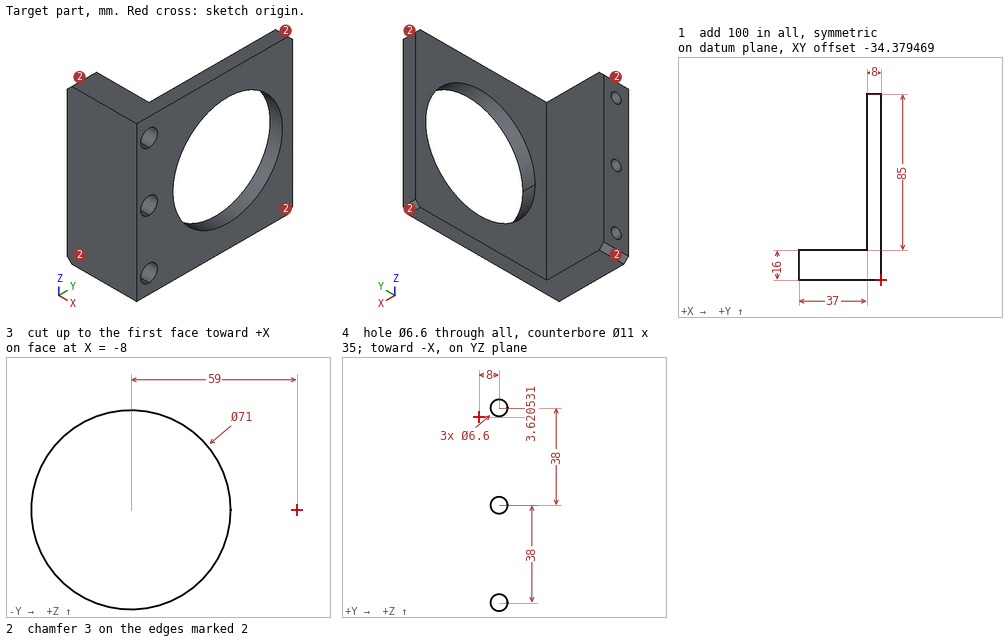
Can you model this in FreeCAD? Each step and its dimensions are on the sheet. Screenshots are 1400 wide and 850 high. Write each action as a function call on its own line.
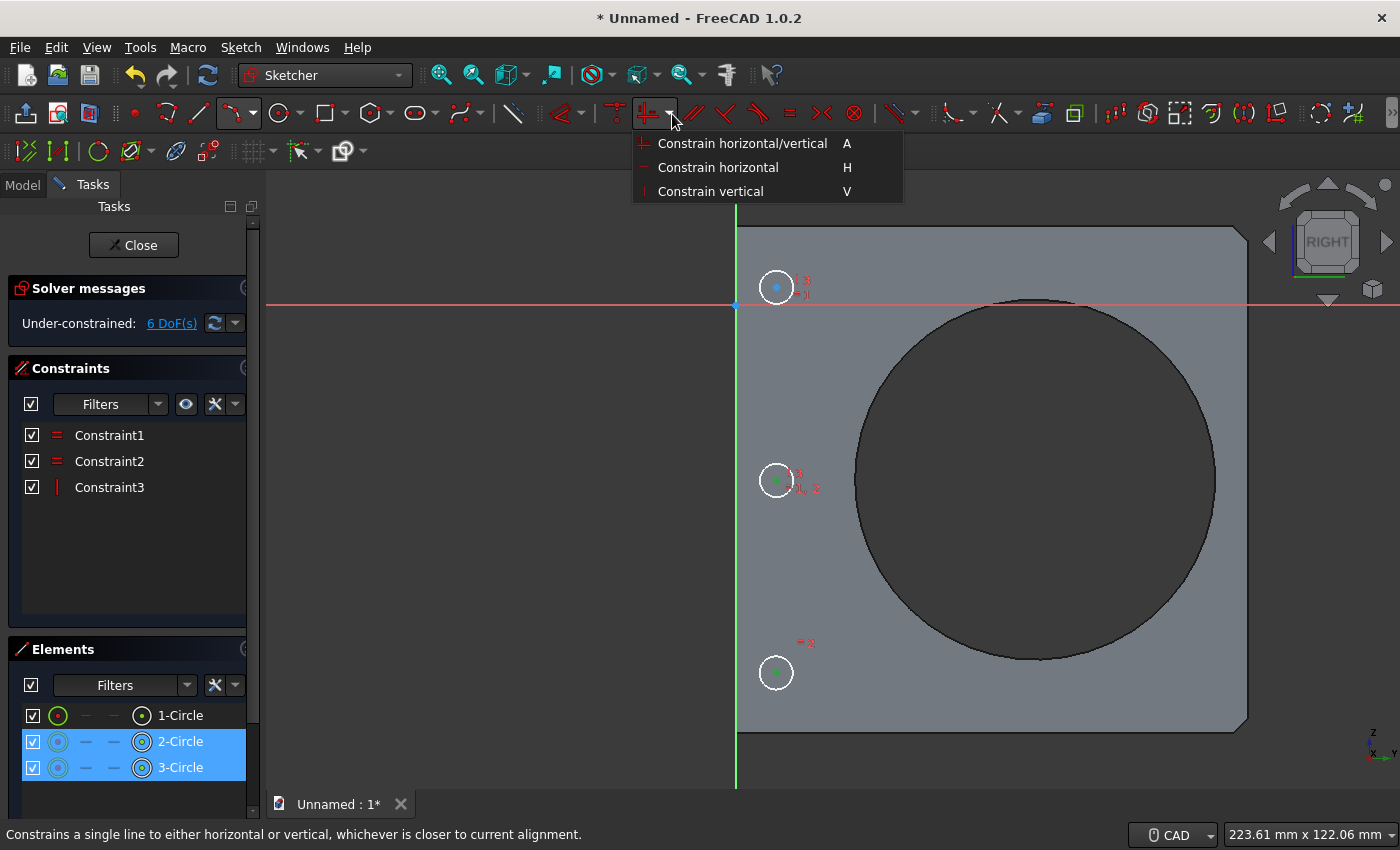
click(768, 191)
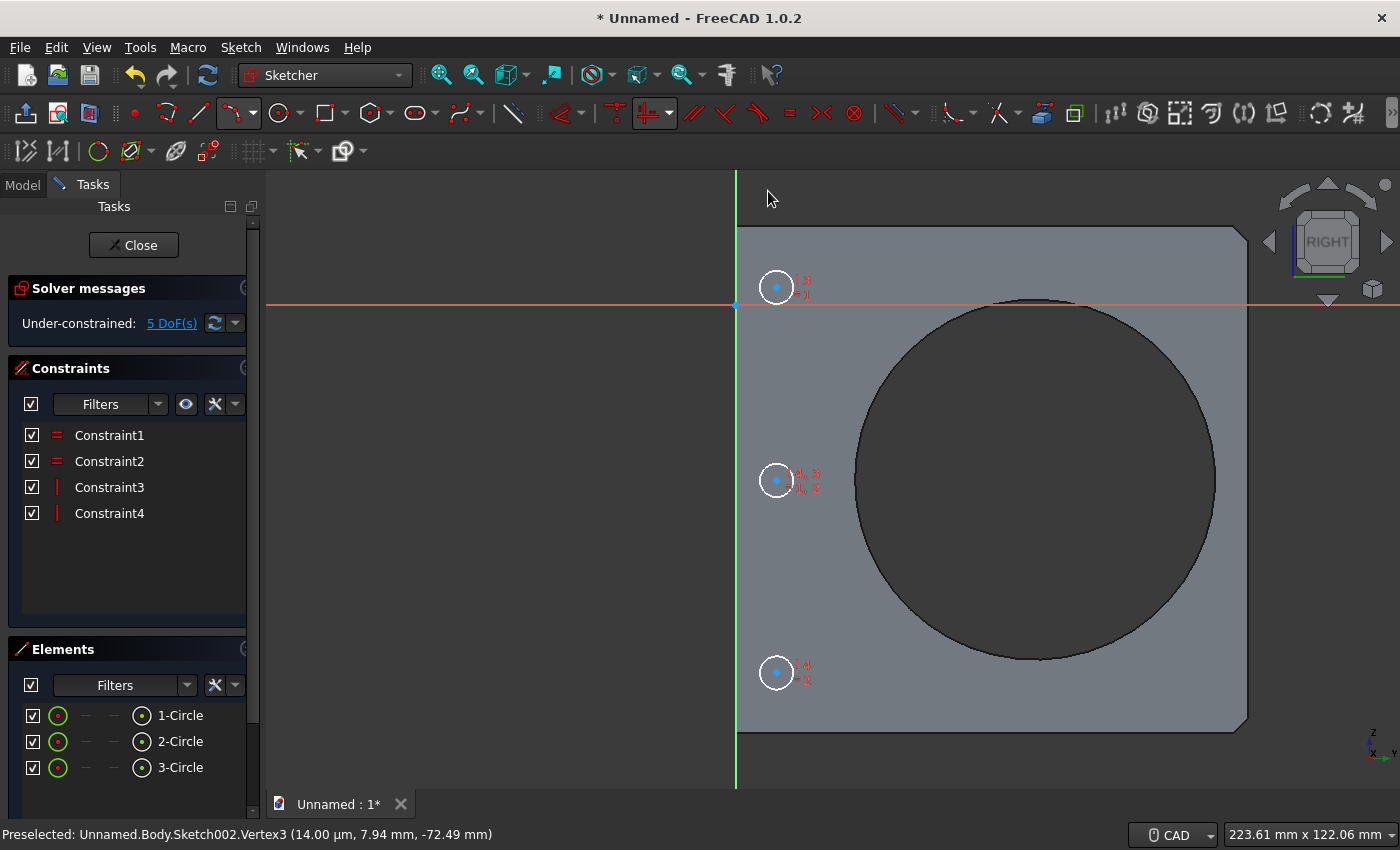
click(560, 114)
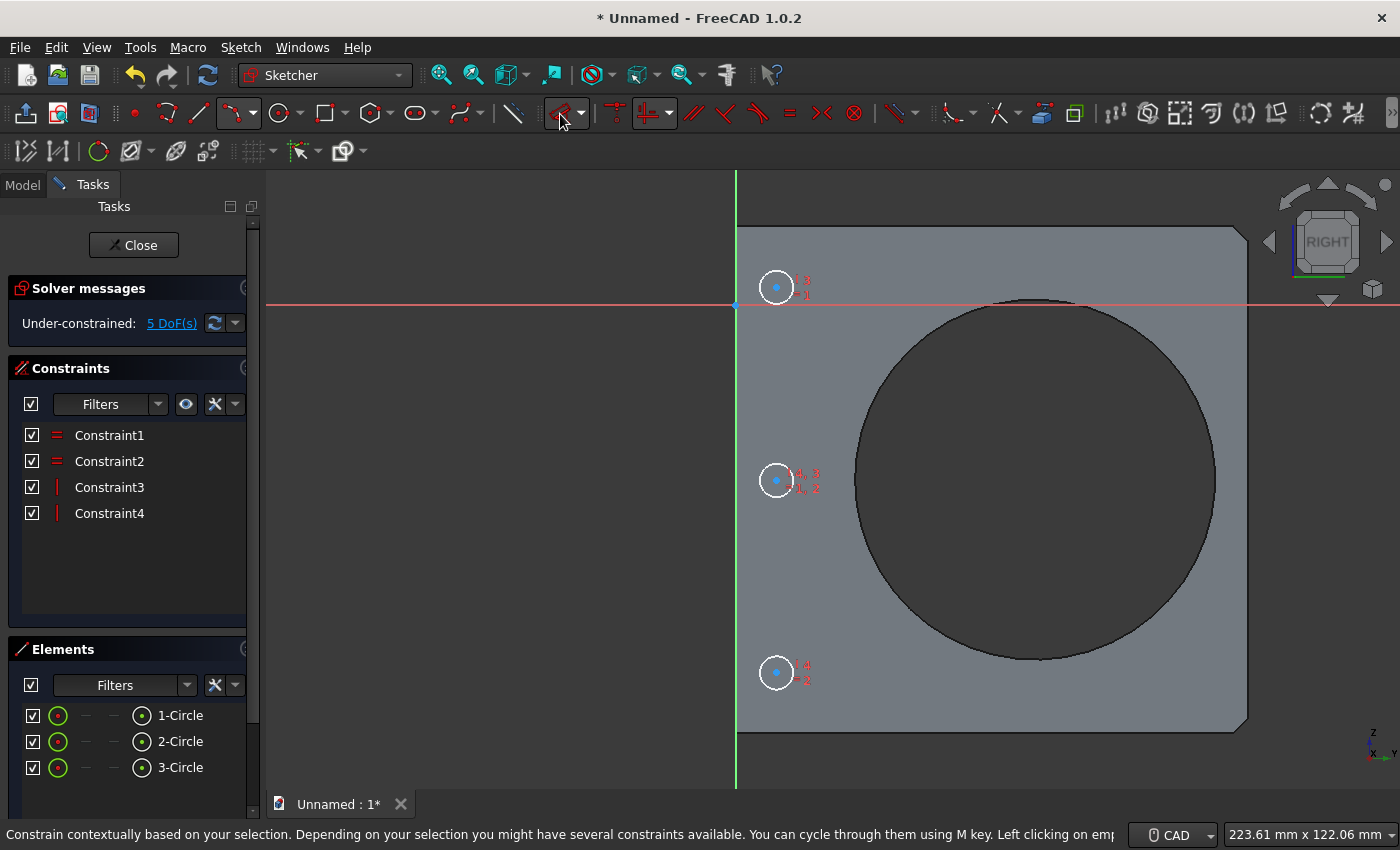
click(788, 276)
click(811, 253)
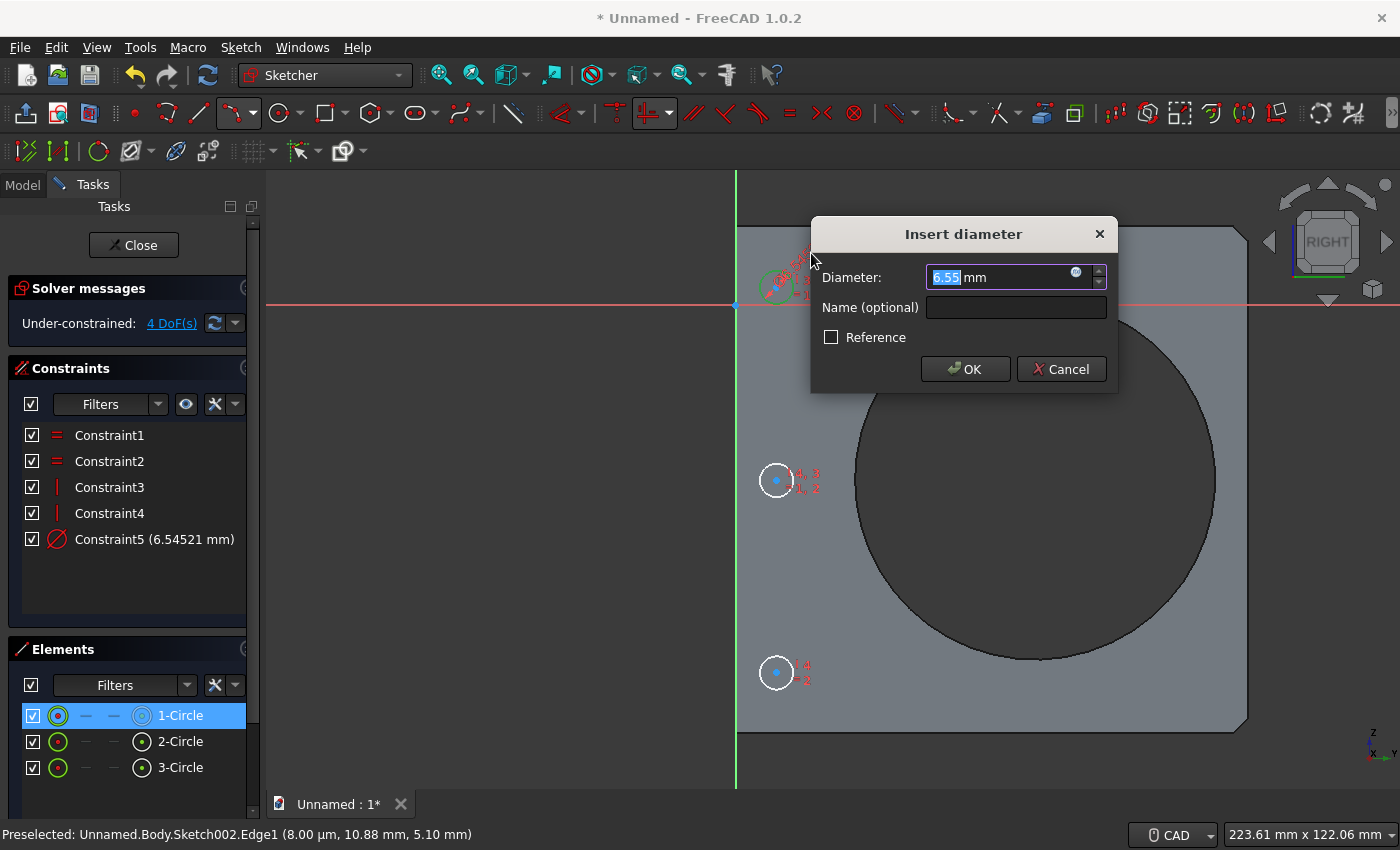
text(6.6)
key(Return)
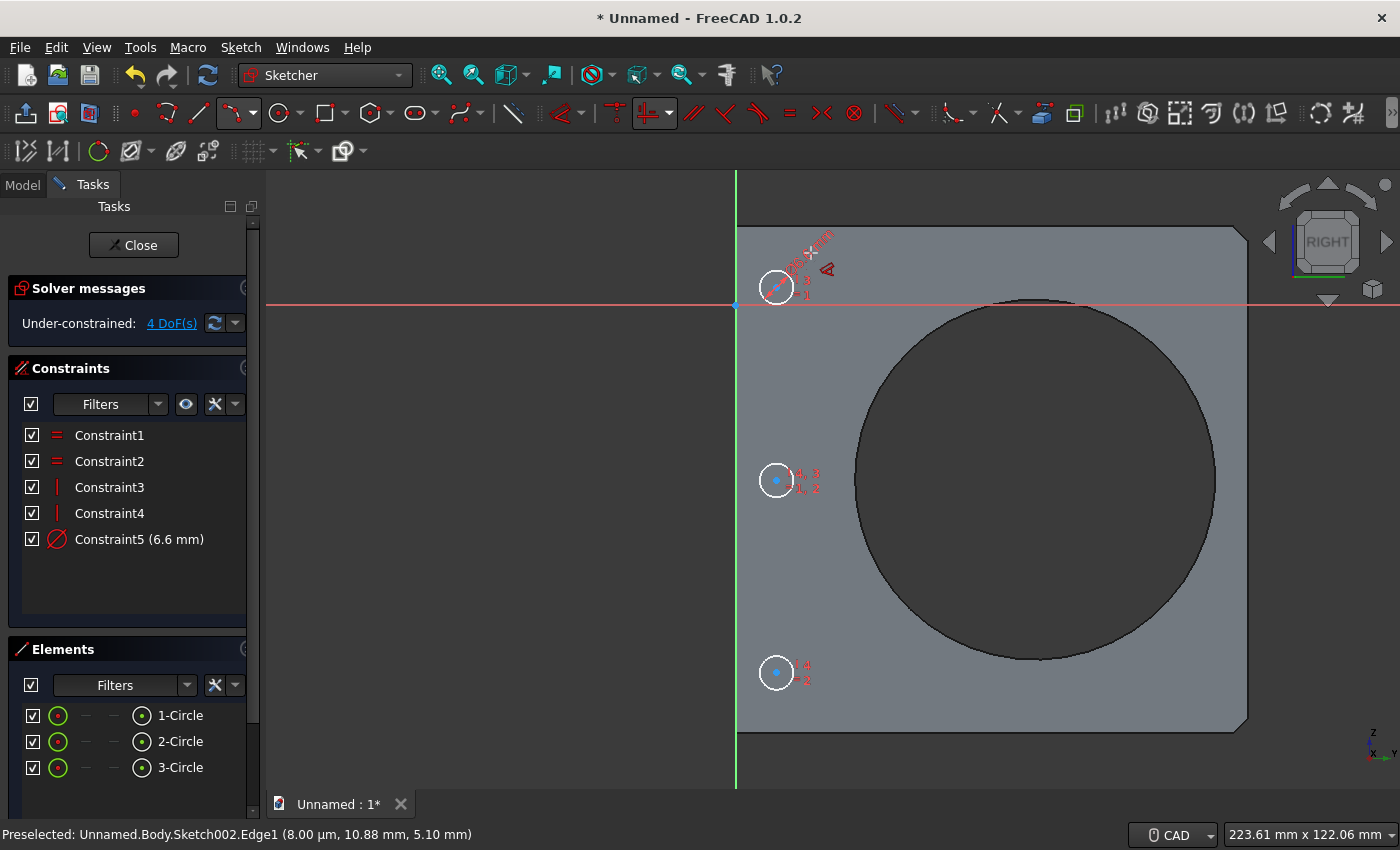
click(777, 287)
click(756, 339)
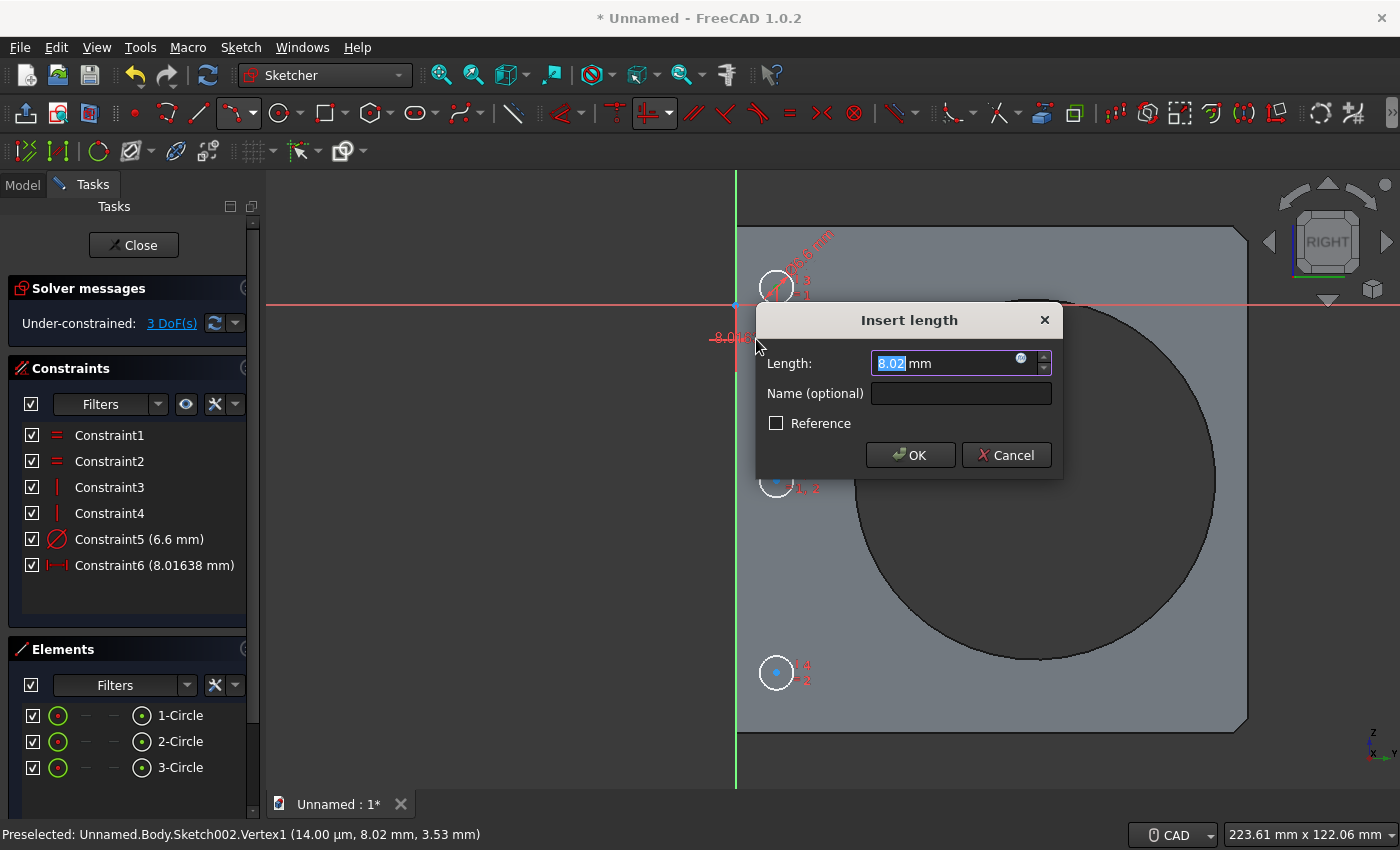
text(8)
key(Return)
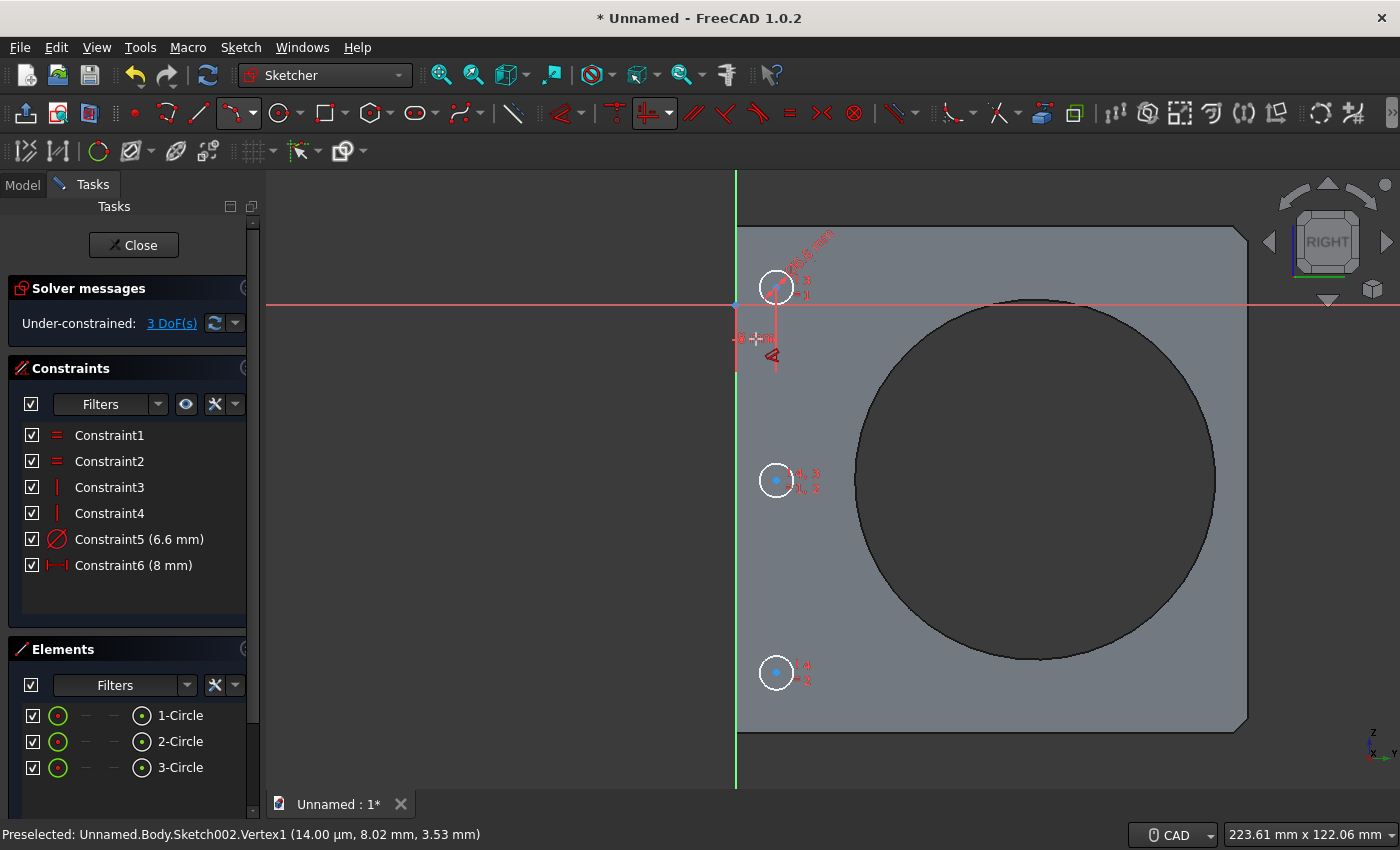
click(776, 287)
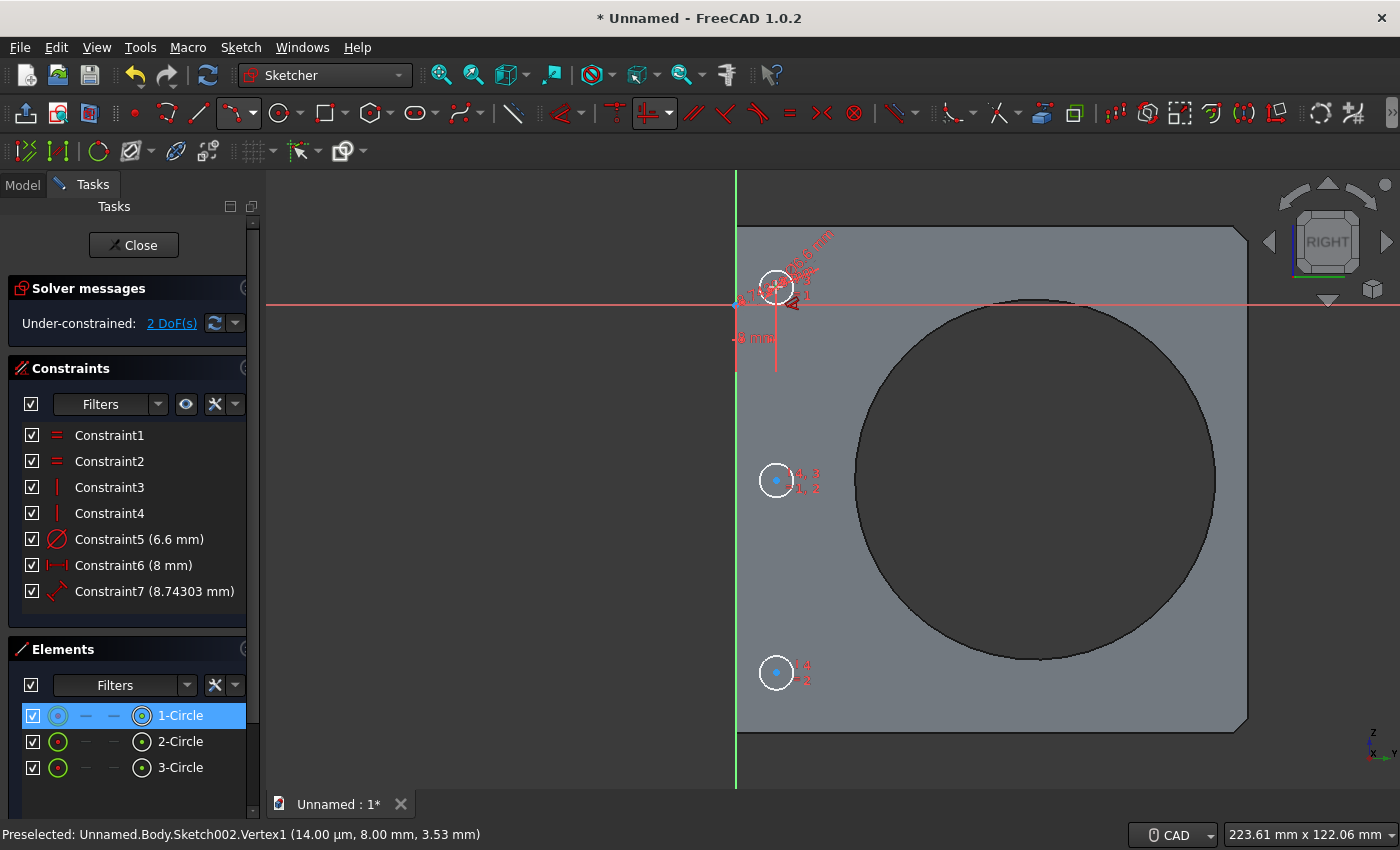
click(776, 480)
click(810, 384)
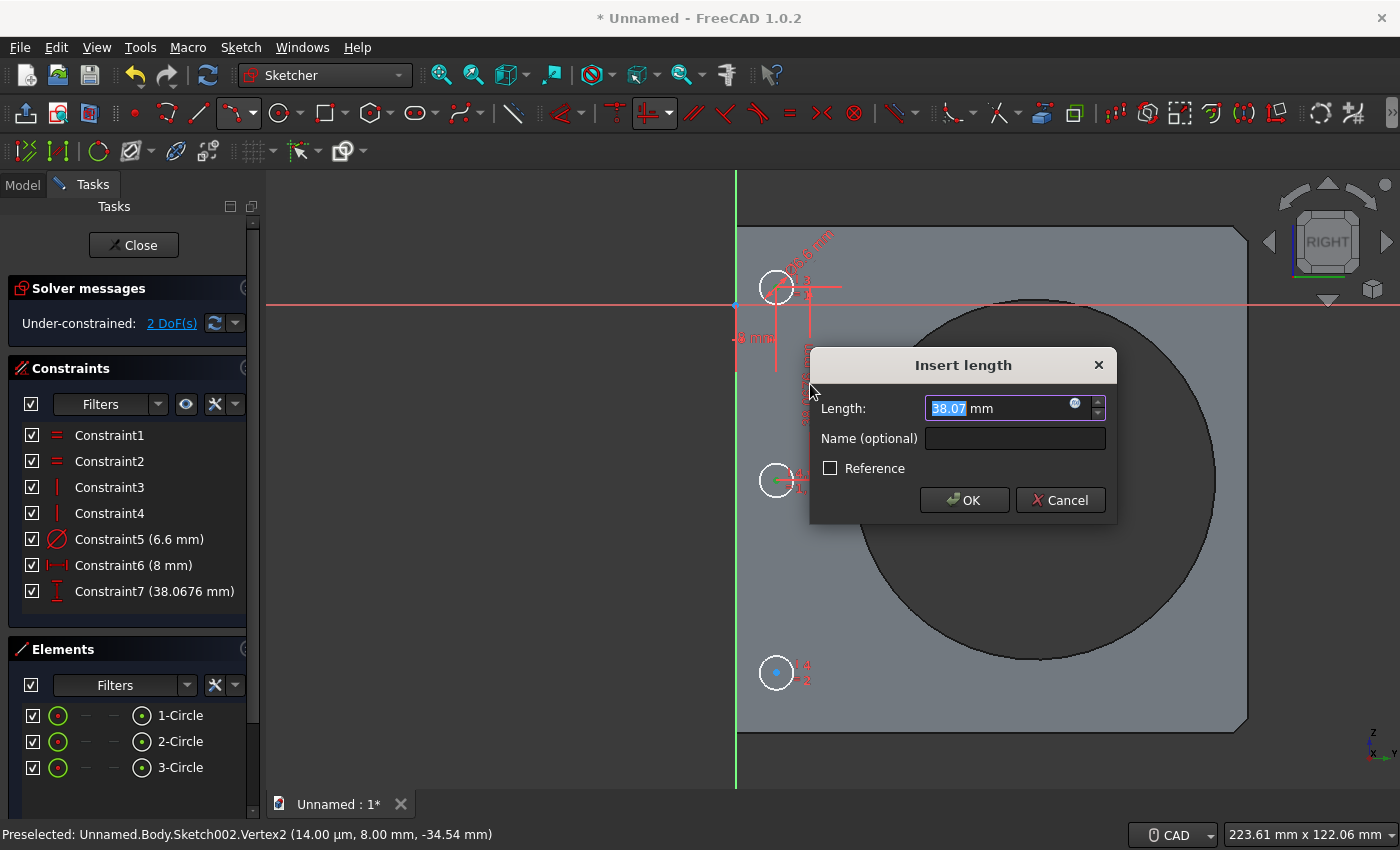
text(38)
key(Return)